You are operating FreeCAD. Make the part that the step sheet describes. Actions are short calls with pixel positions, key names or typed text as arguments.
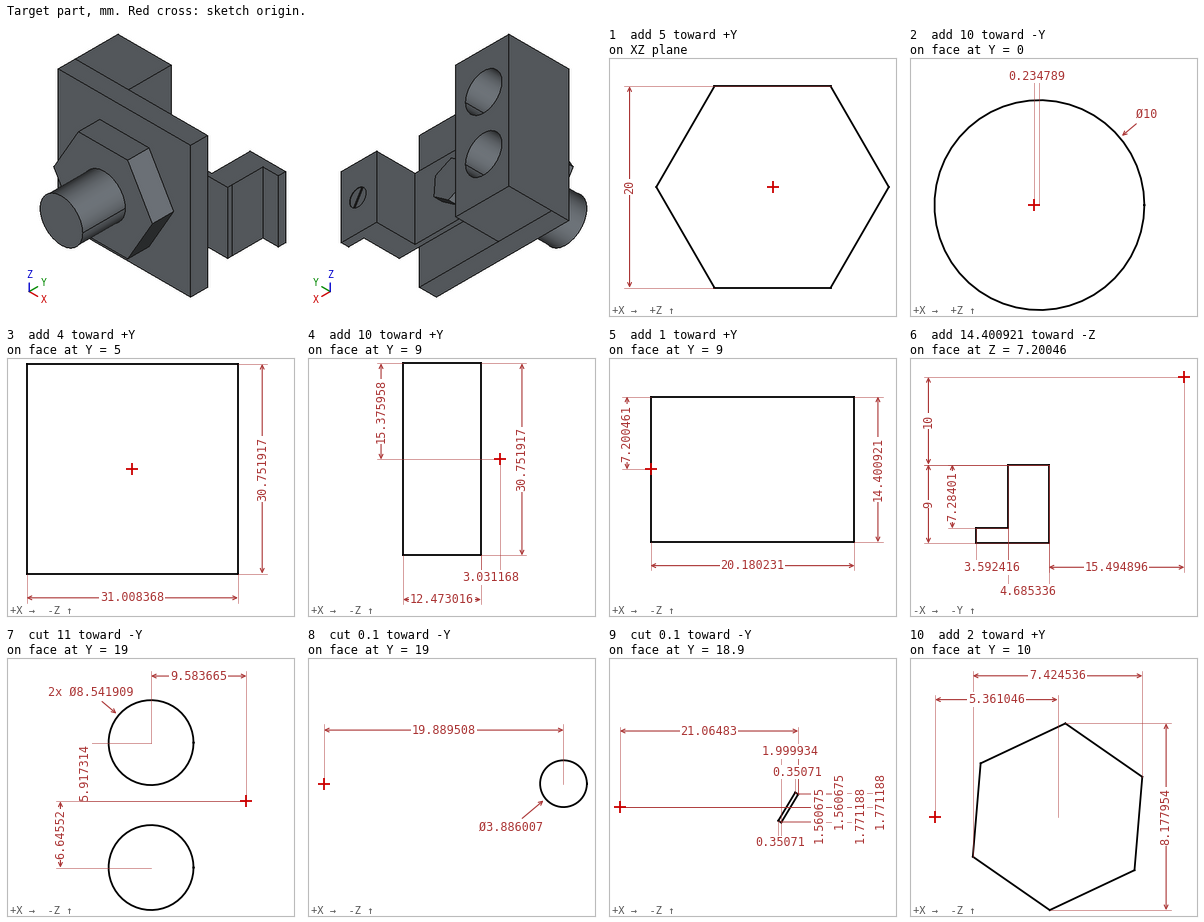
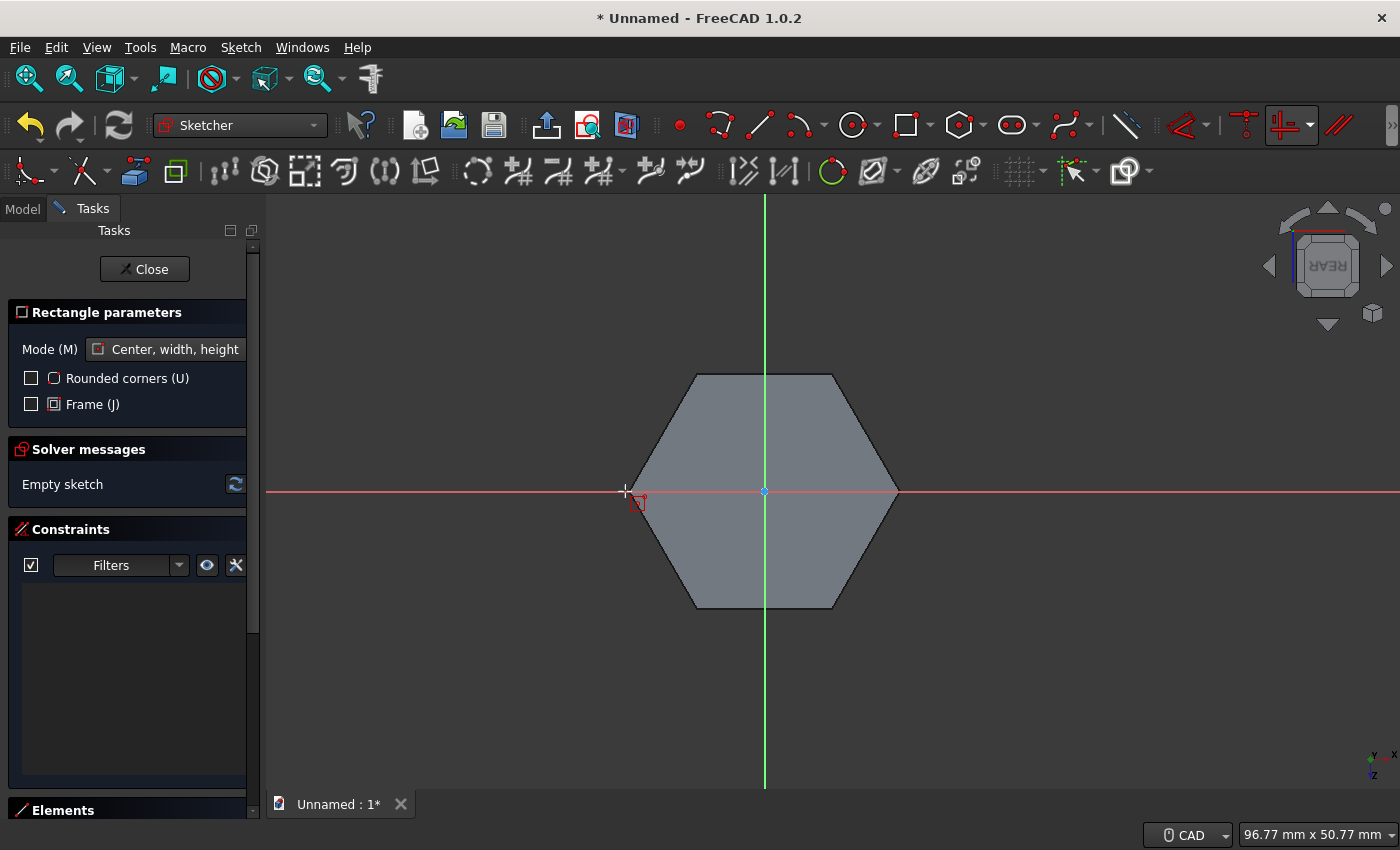
click(765, 492)
move(946, 311)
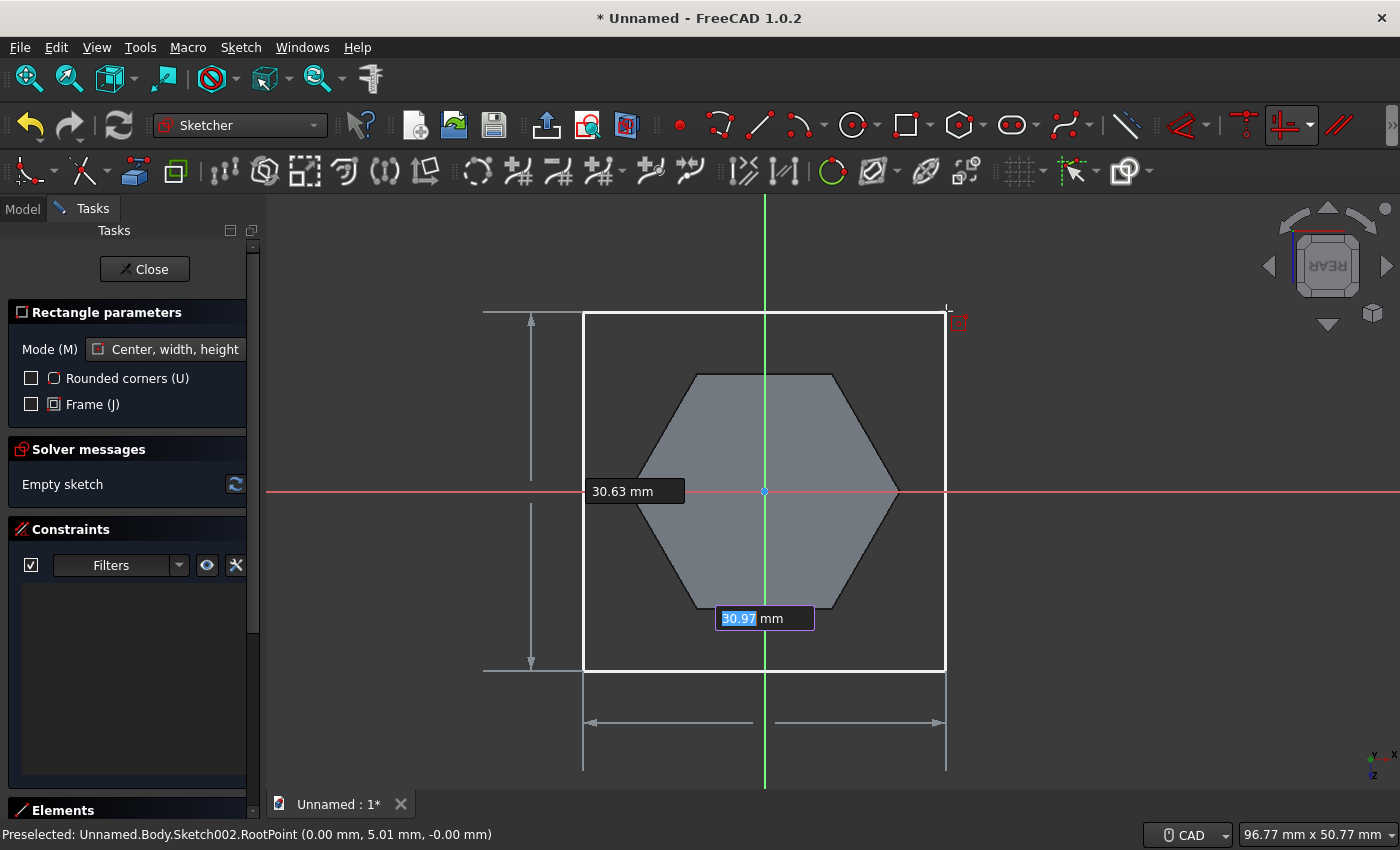
text(31.008368)
key(Tab)
text(30.751917)
key(Return)
key(Escape)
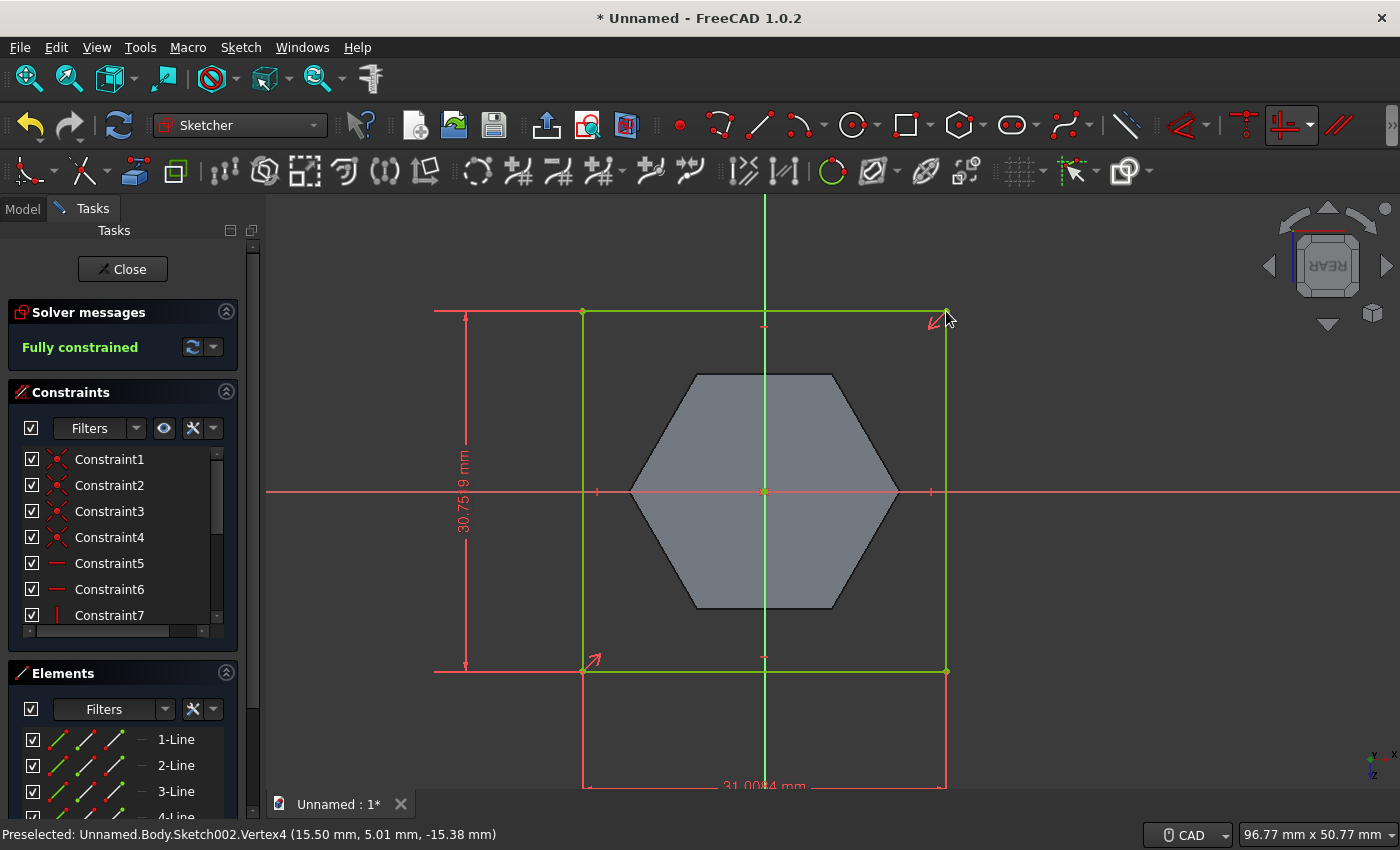
click(123, 269)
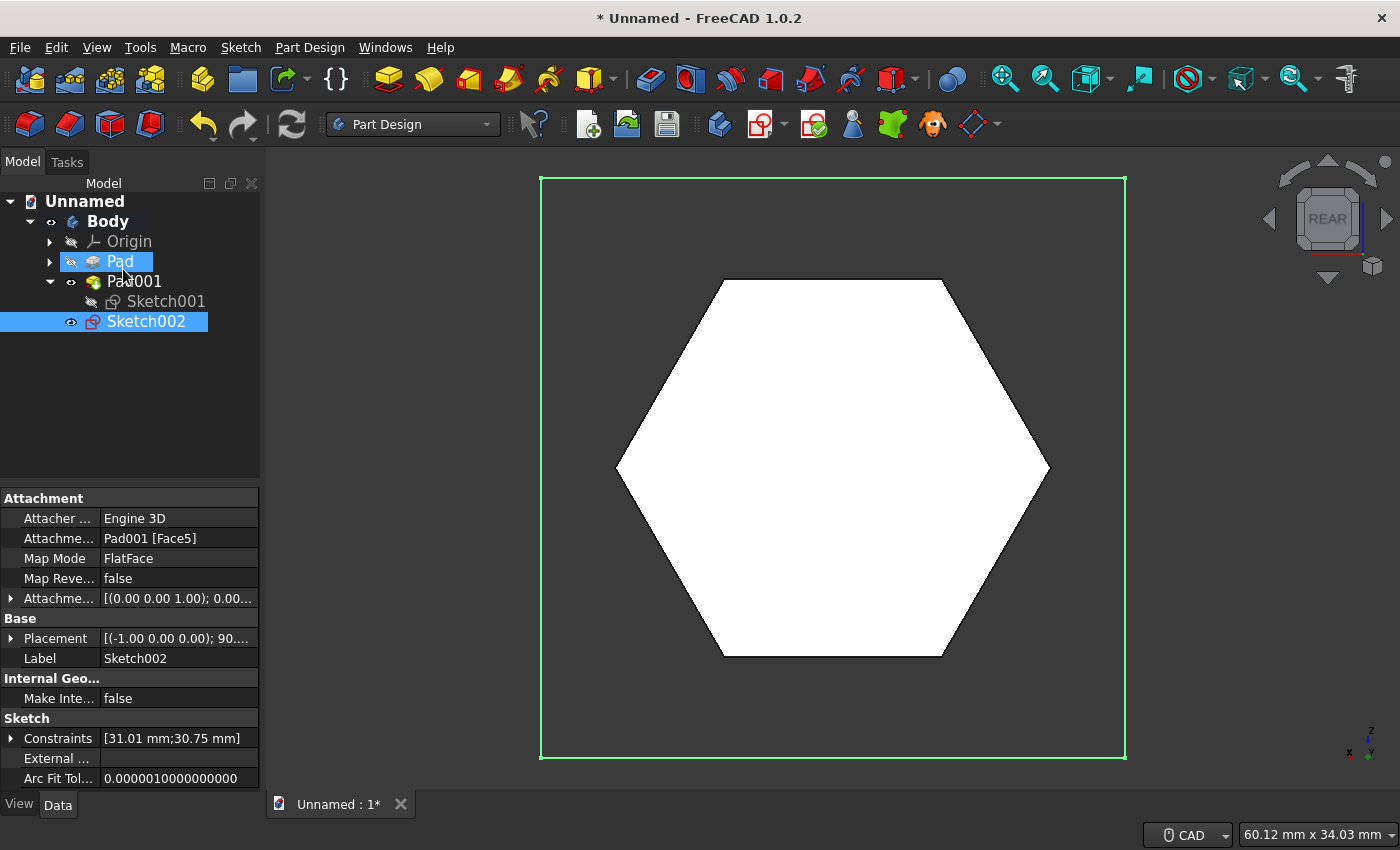
click(390, 80)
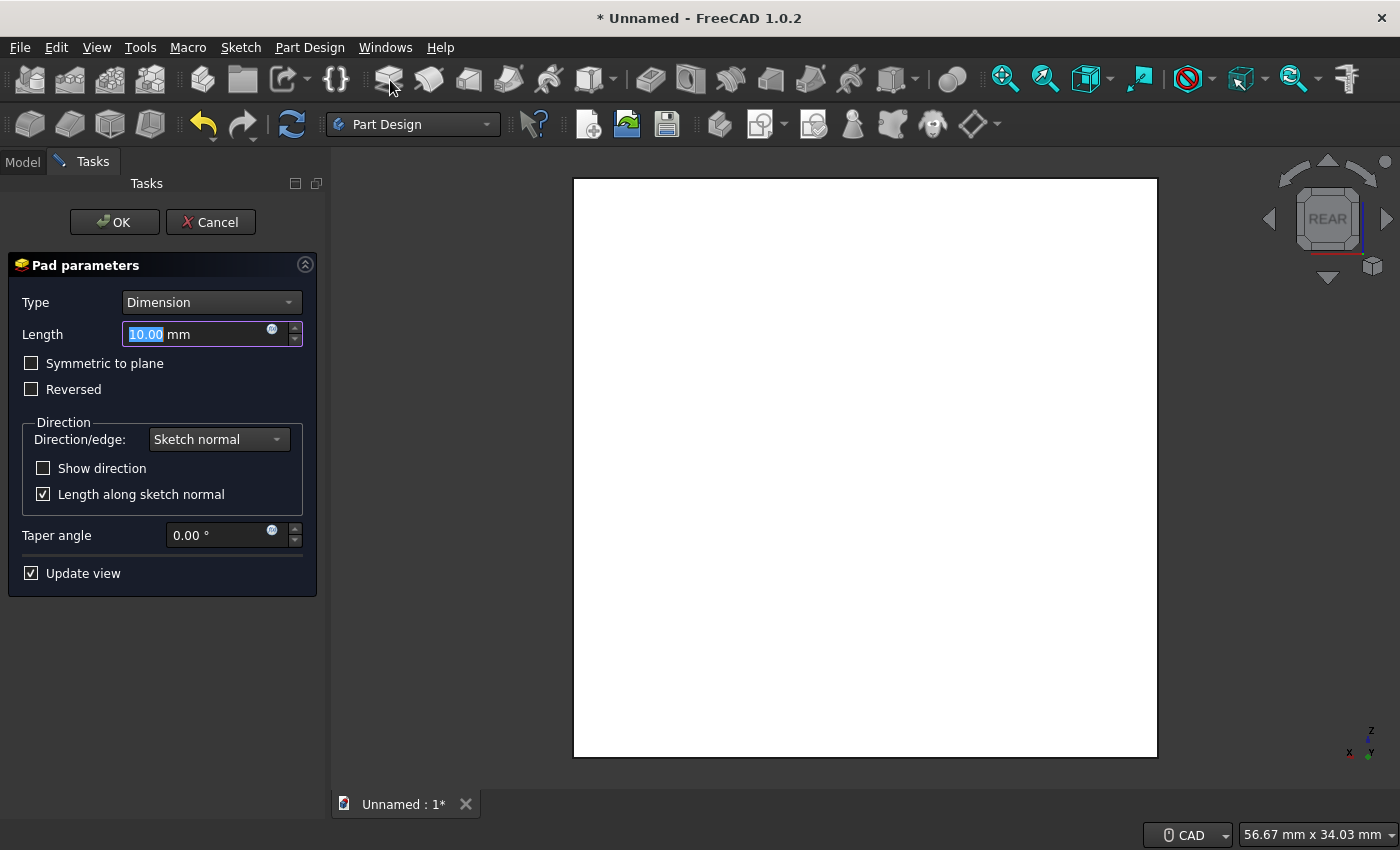
text(4)
key(Tab)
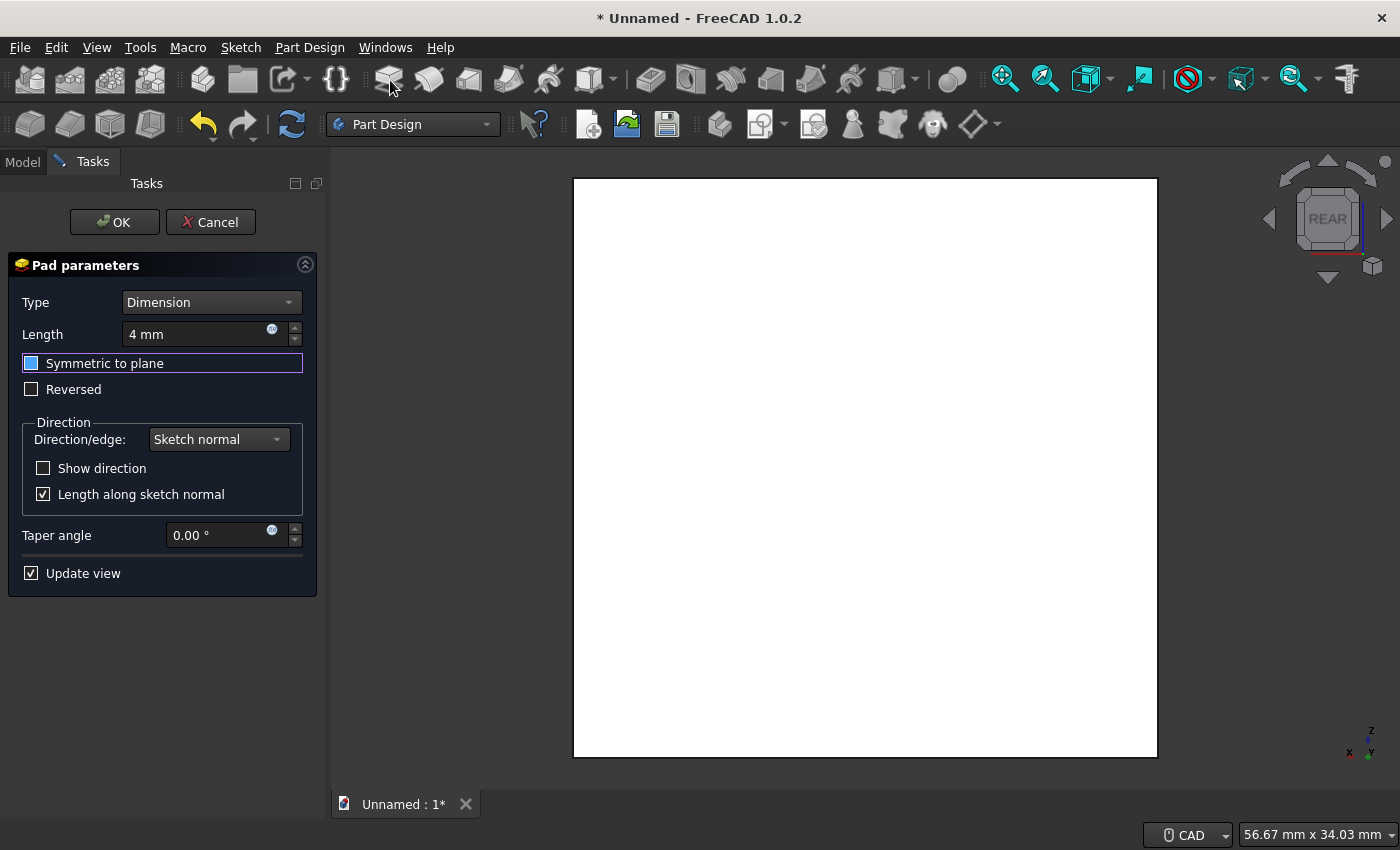
click(115, 222)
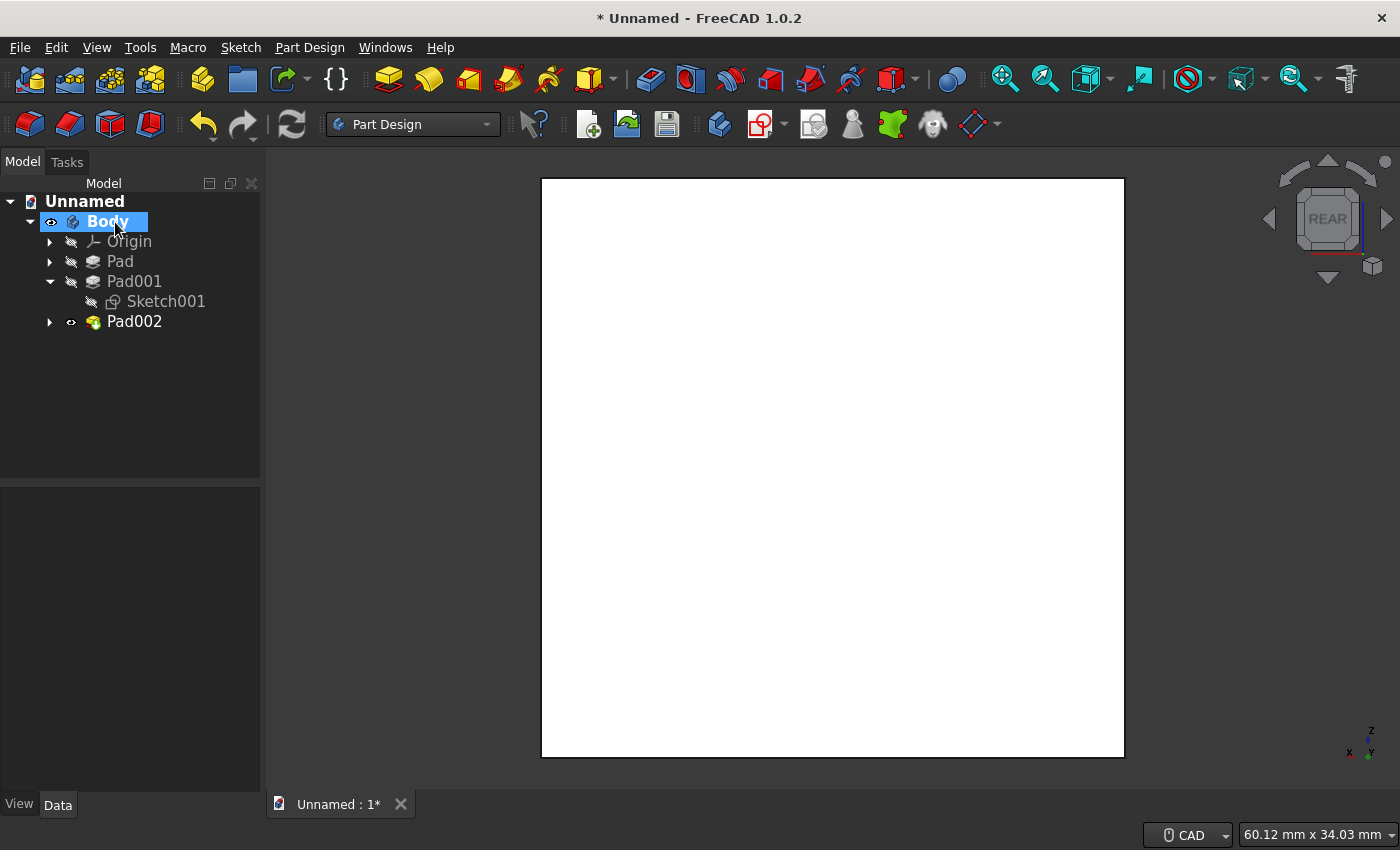
click(833, 467)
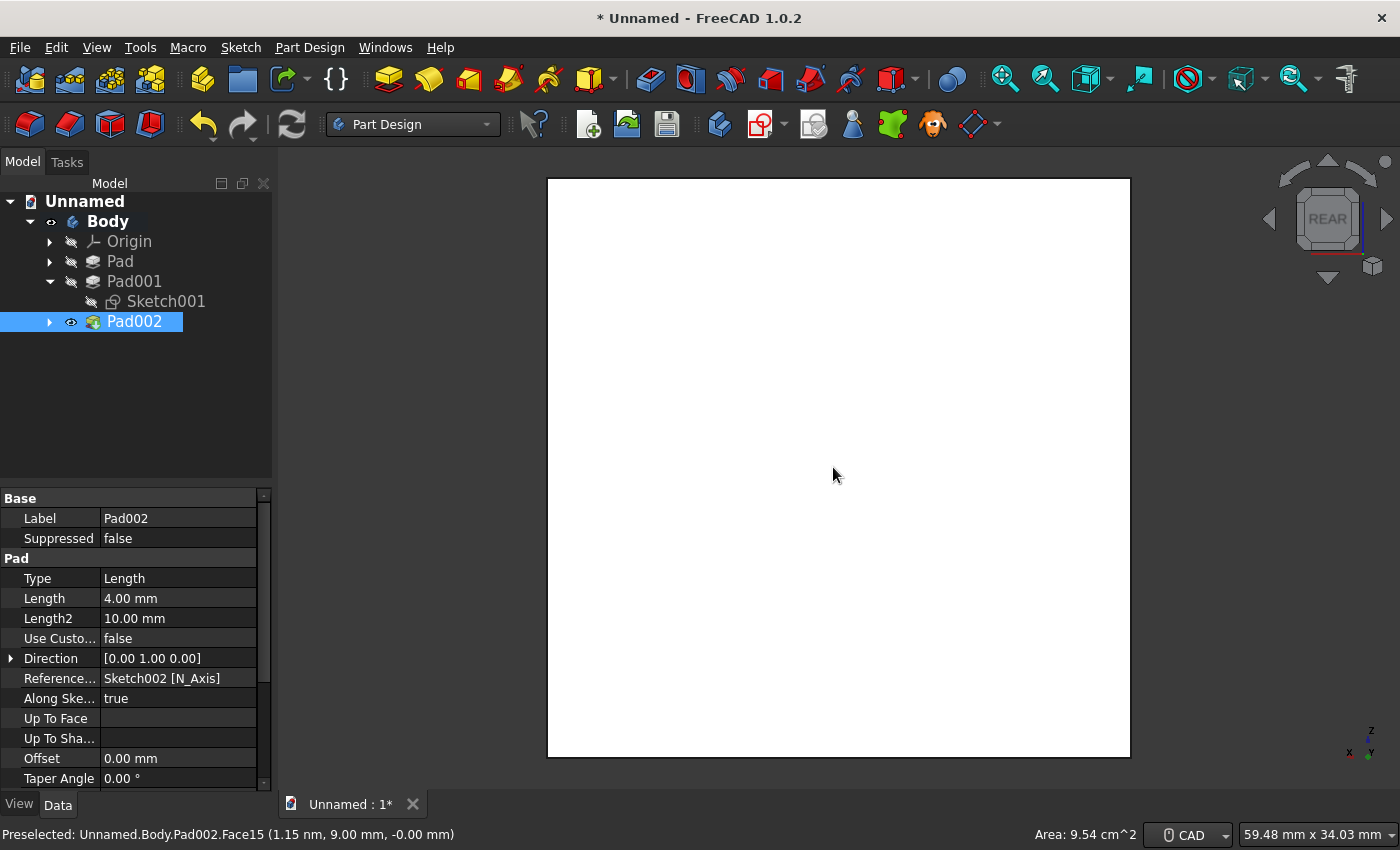
click(760, 124)